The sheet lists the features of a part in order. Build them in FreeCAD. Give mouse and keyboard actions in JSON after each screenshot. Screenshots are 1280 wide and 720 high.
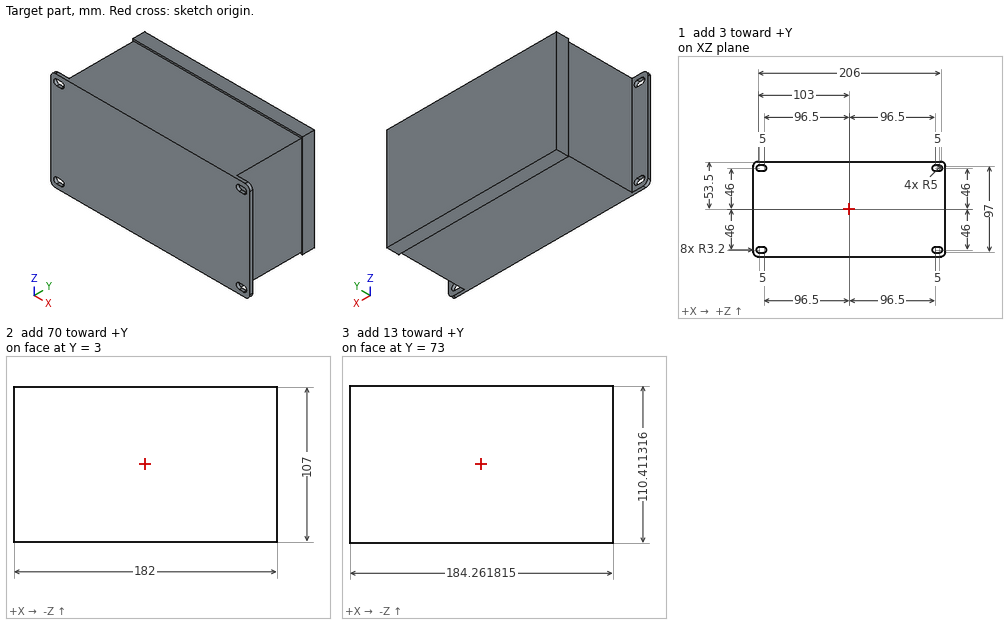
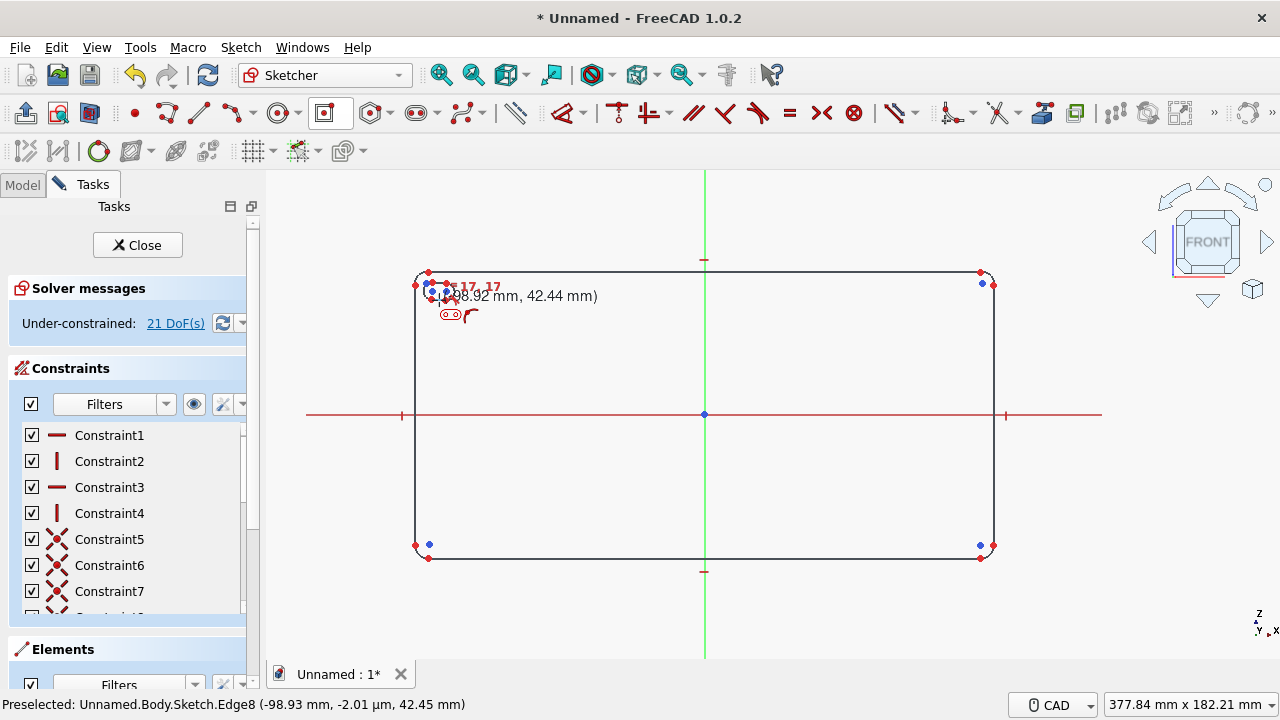
{"action": "scroll", "coordinate": [964, 291], "scroll_direction": "up", "scroll_amount": 5}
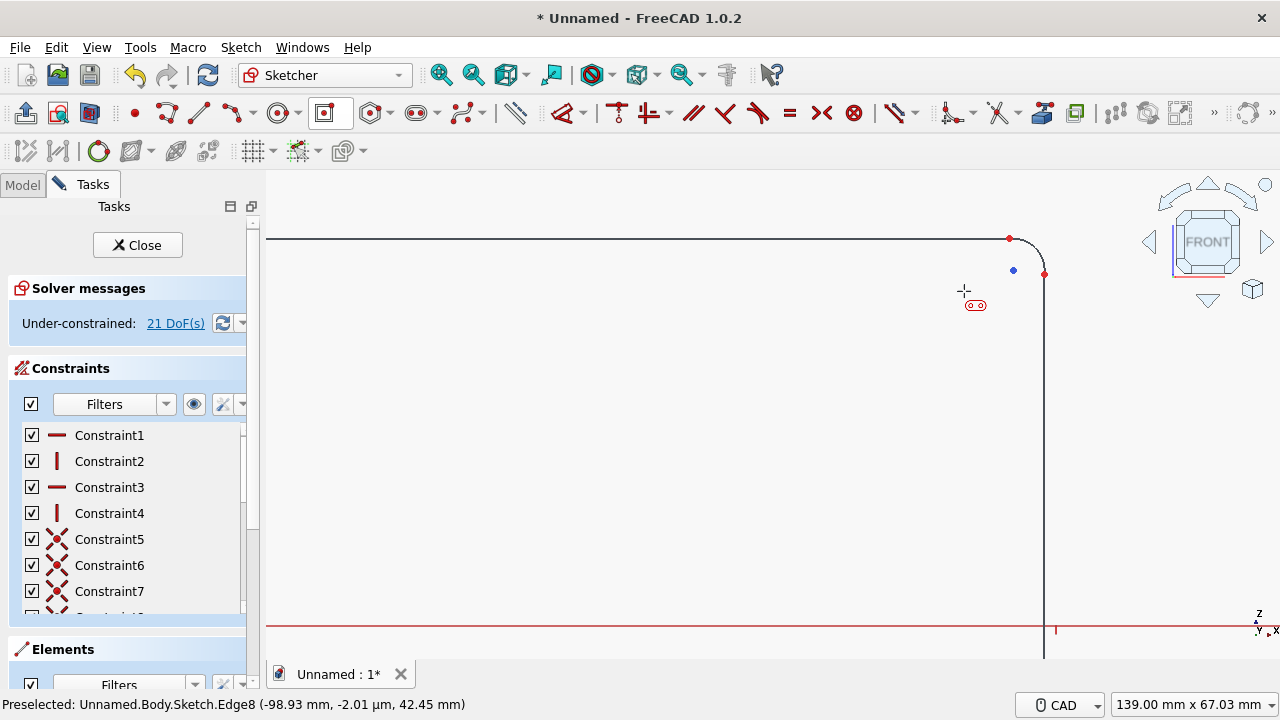
{"action": "left_click", "coordinate": [962, 291]}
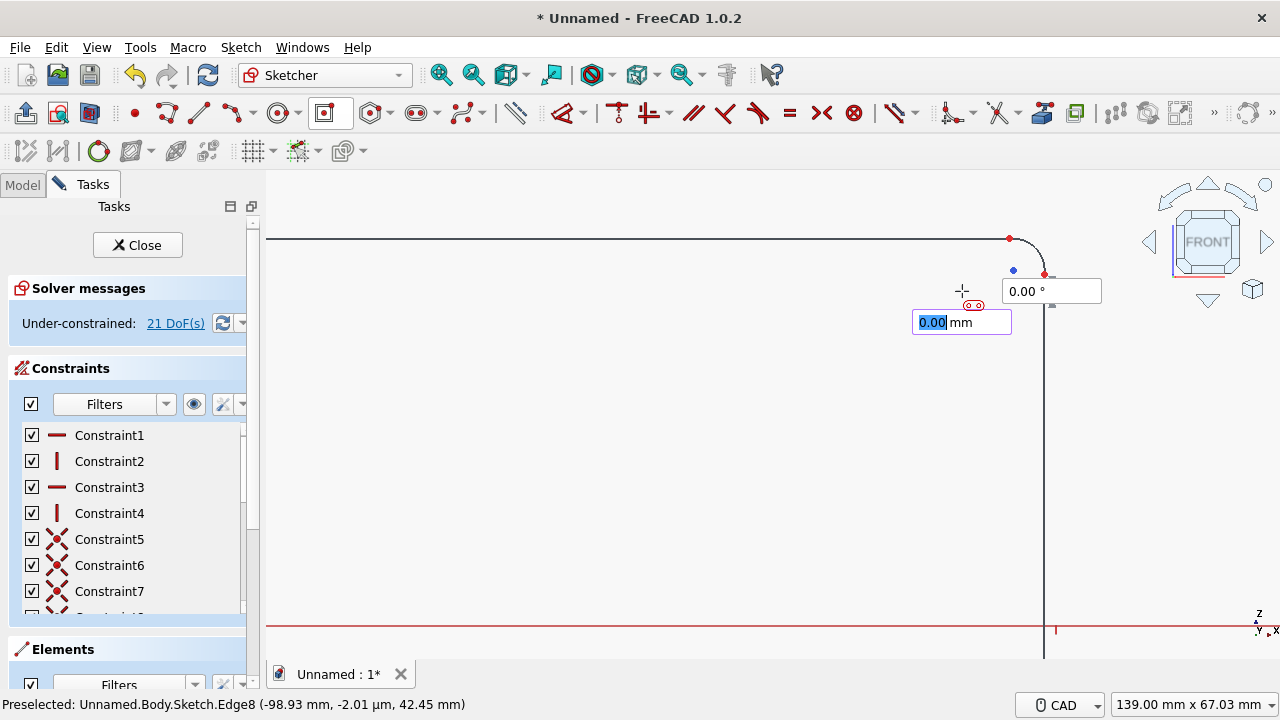
{"action": "left_click", "coordinate": [998, 291]}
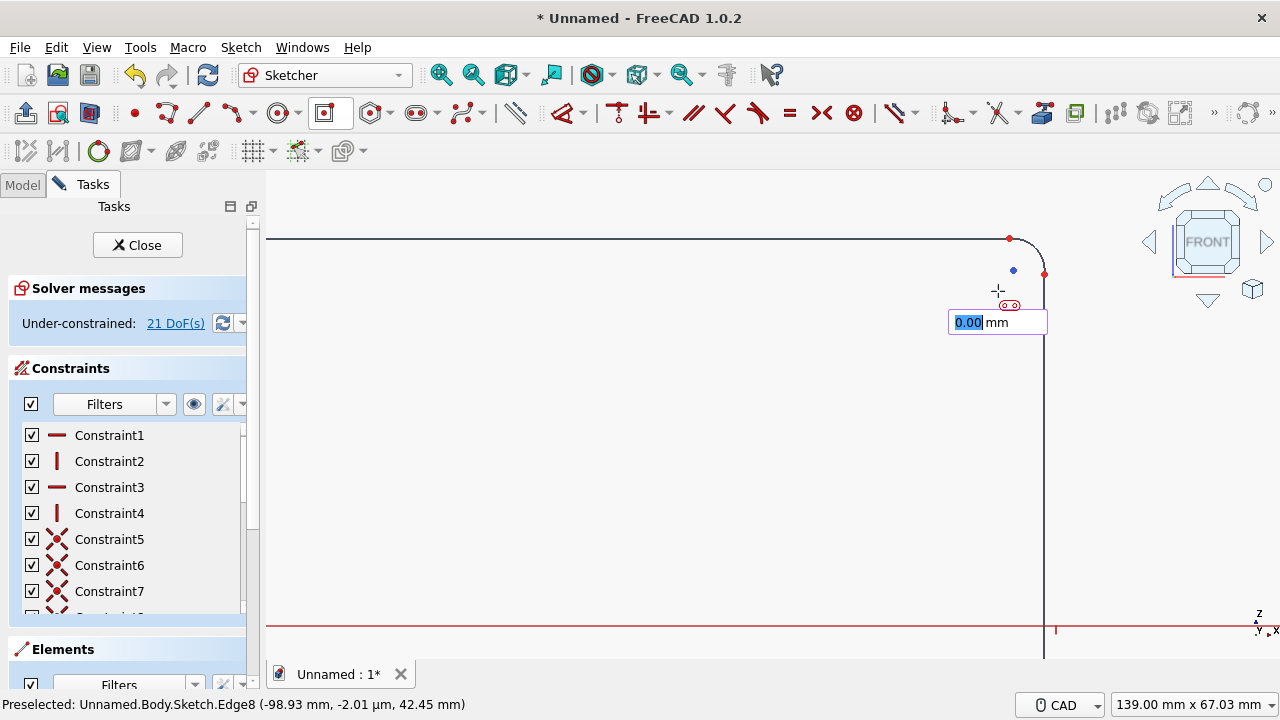
{"action": "left_click", "coordinate": [980, 314]}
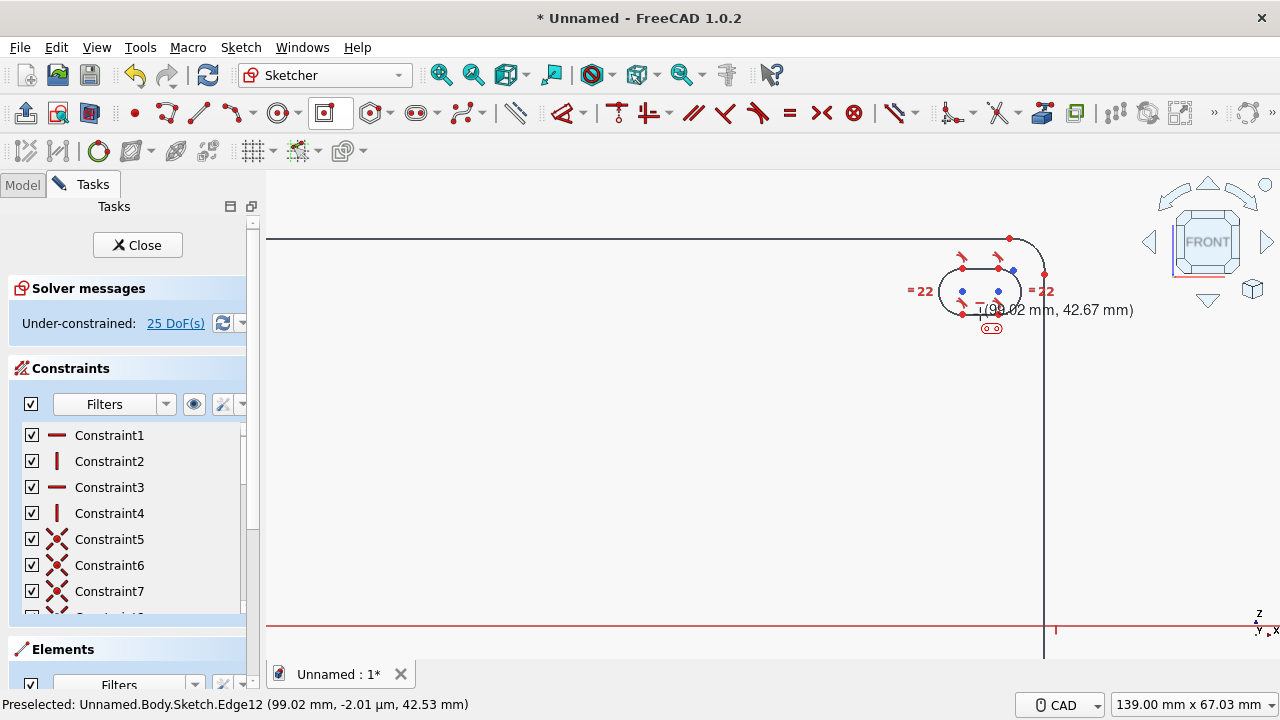
{"action": "scroll", "coordinate": [965, 291], "scroll_direction": "down", "scroll_amount": 5}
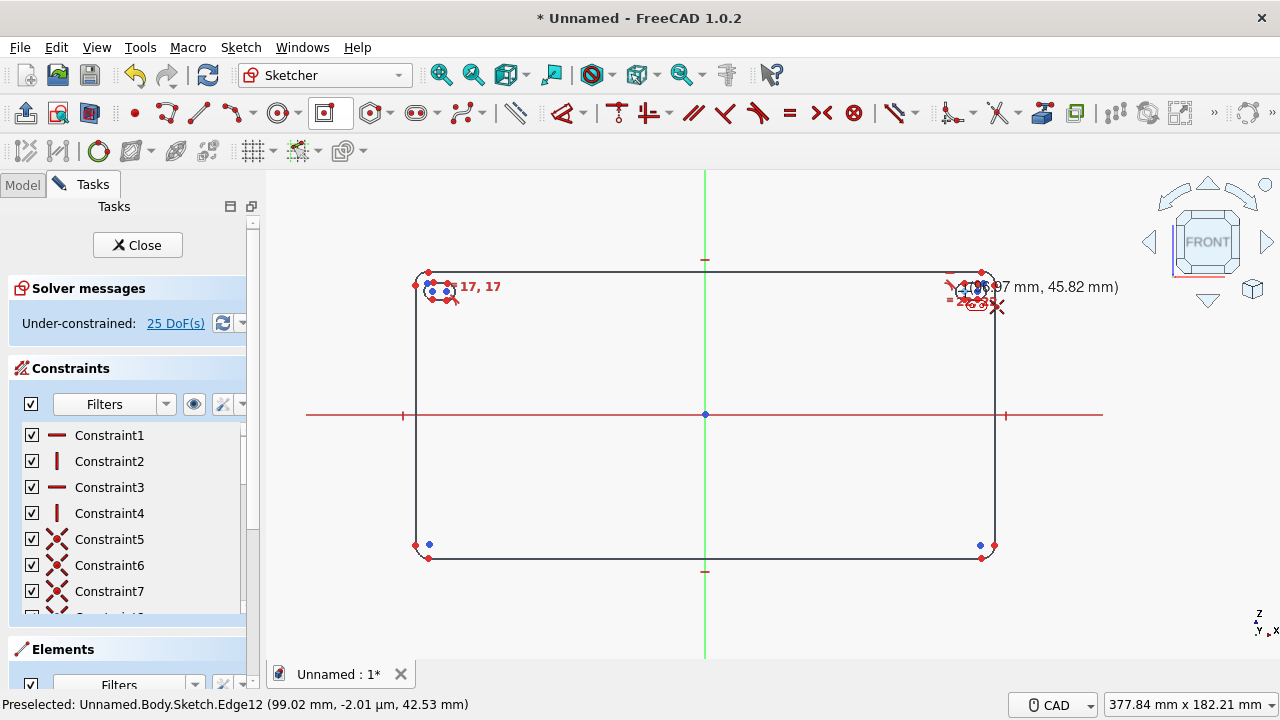
{"action": "scroll", "coordinate": [433, 538], "scroll_direction": "up", "scroll_amount": 5}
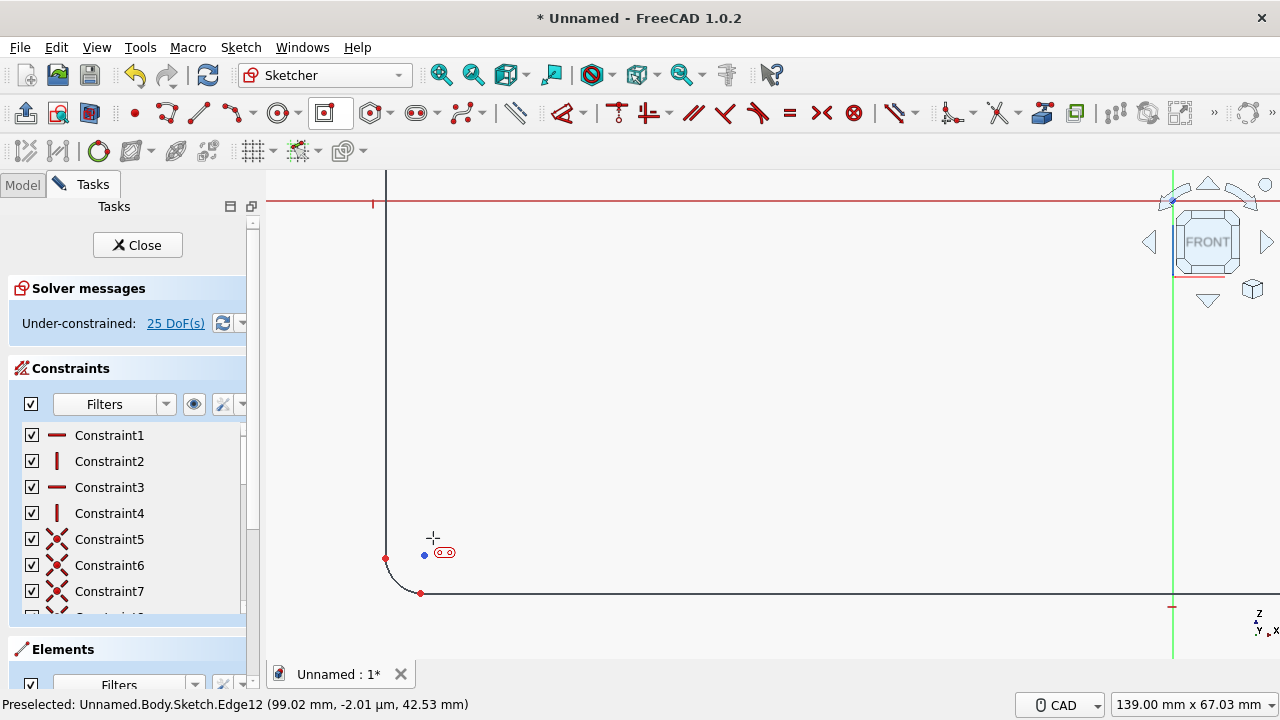
{"action": "left_click", "coordinate": [432, 537]}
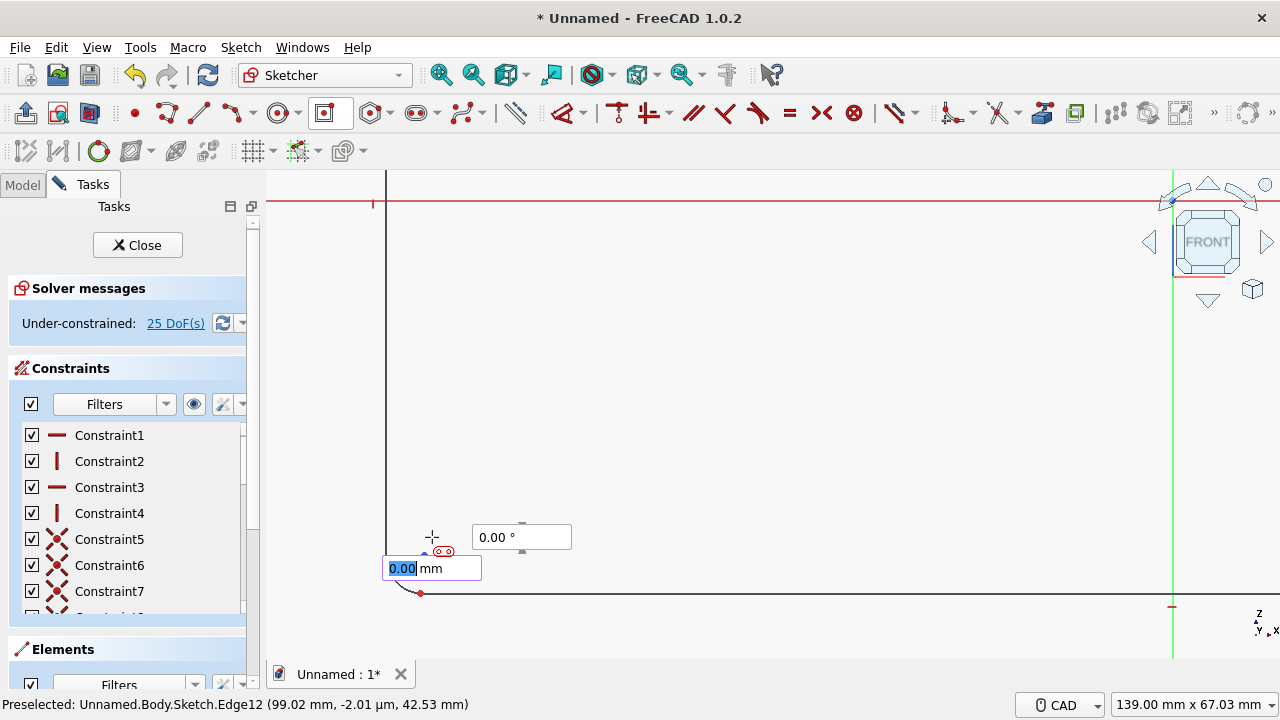
{"action": "left_click", "coordinate": [469, 537]}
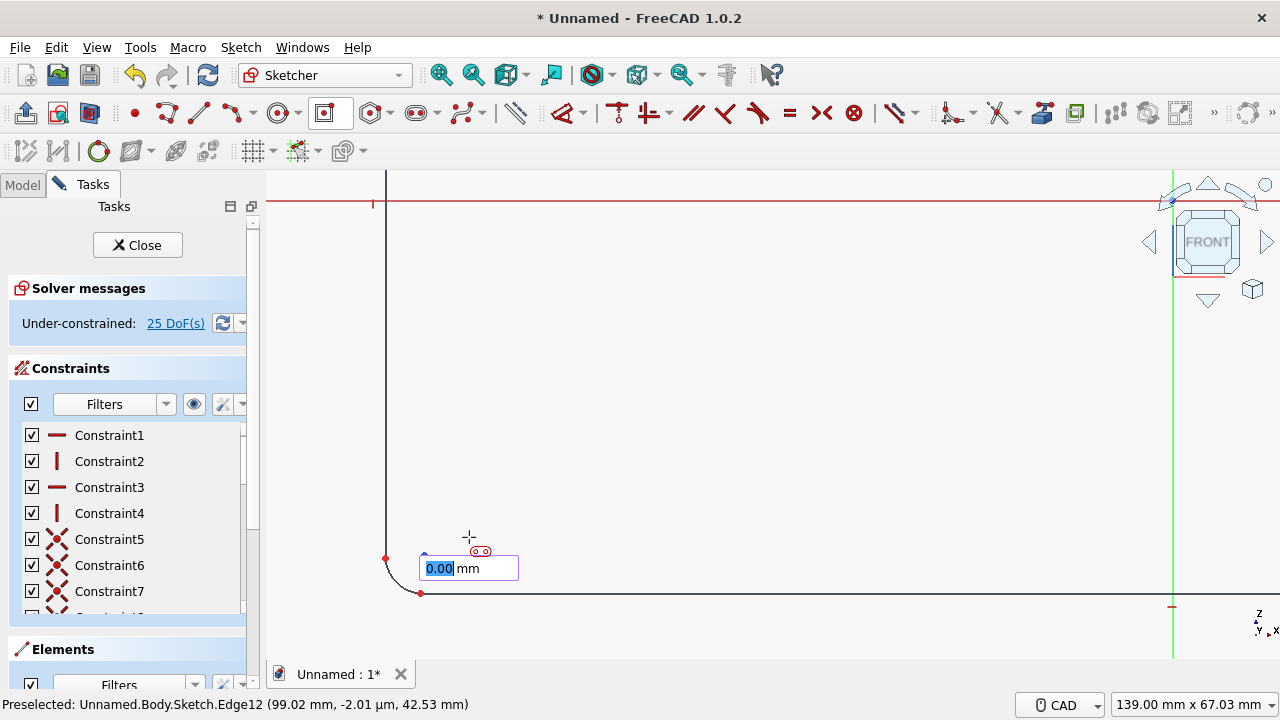
{"action": "left_click", "coordinate": [450, 560]}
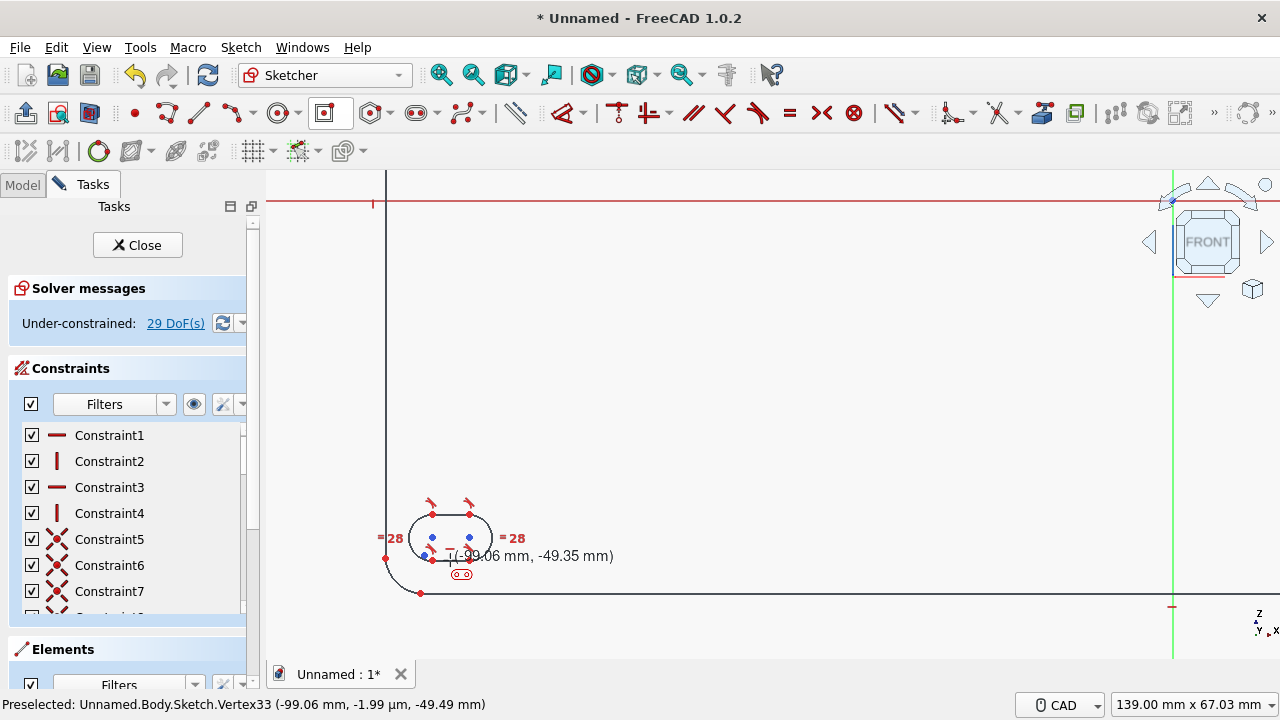
{"action": "scroll", "coordinate": [432, 539], "scroll_direction": "down", "scroll_amount": 5}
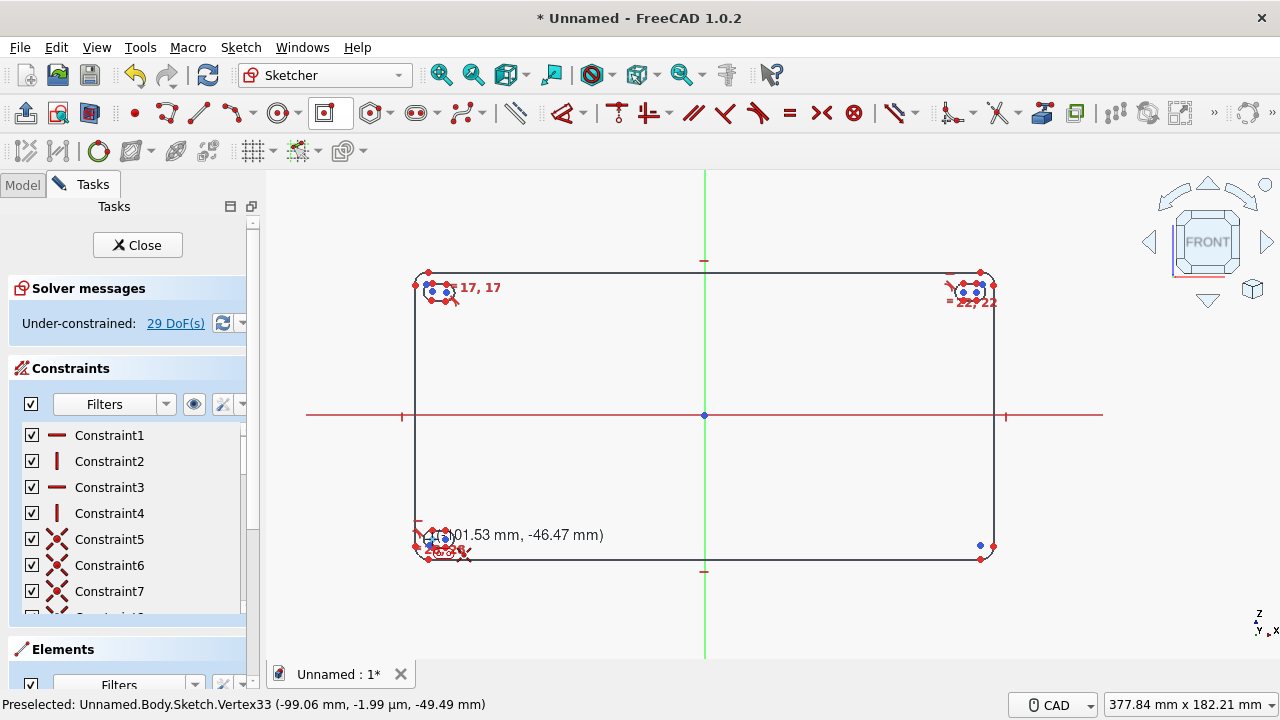
{"action": "scroll", "coordinate": [964, 539], "scroll_direction": "up", "scroll_amount": 5}